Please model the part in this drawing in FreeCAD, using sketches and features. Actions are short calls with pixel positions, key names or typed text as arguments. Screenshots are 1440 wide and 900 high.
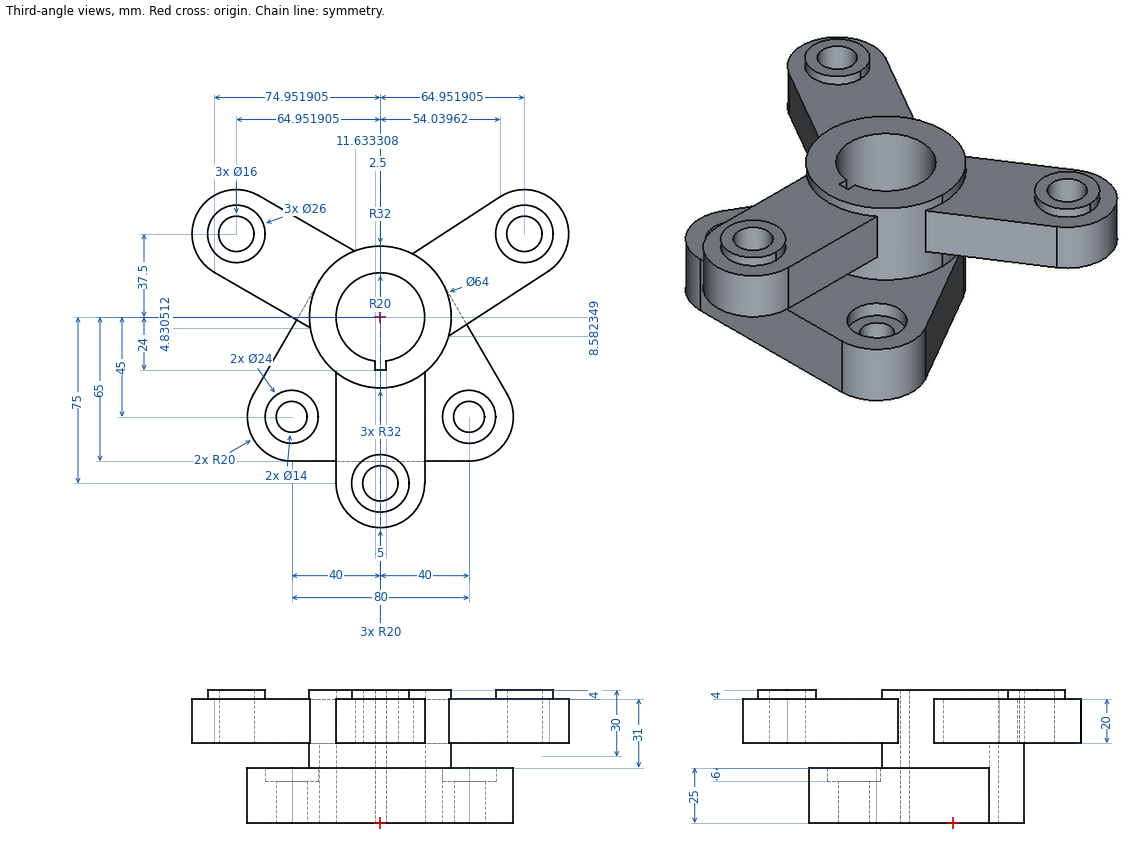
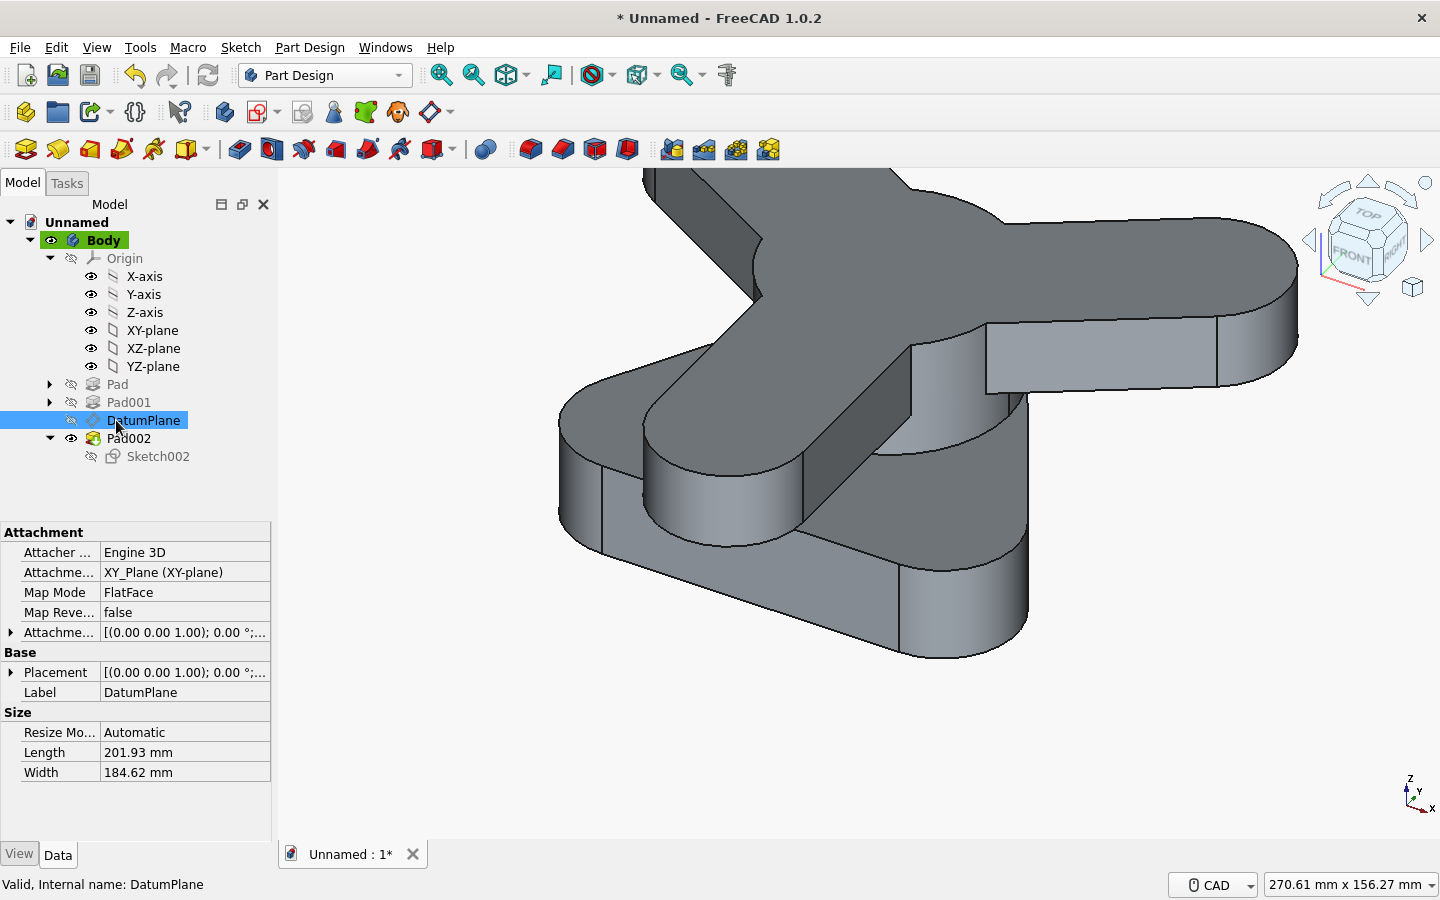
key(v)
key(f)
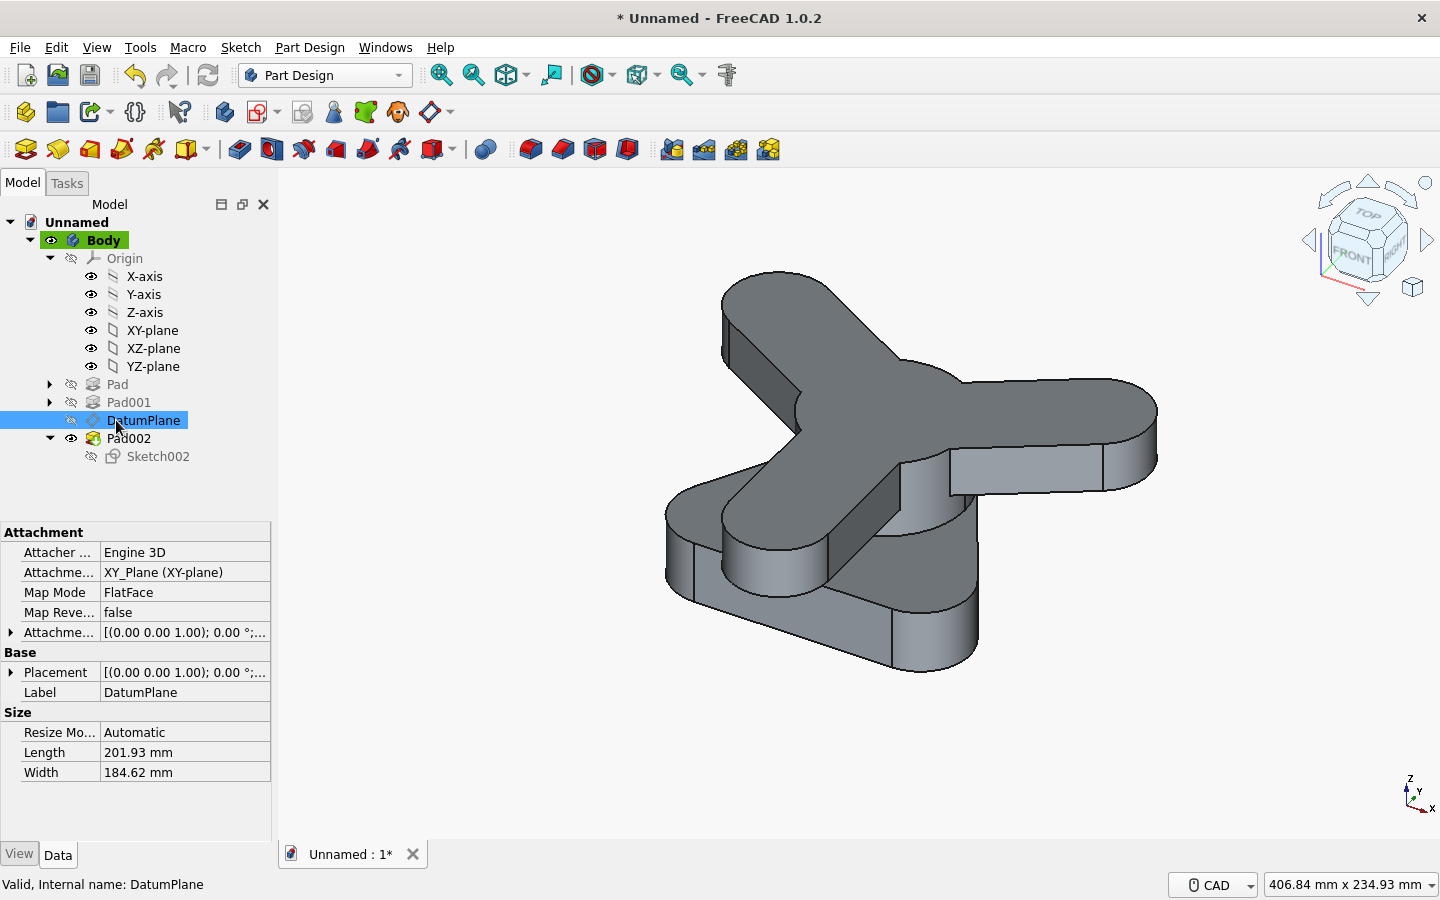
click(890, 406)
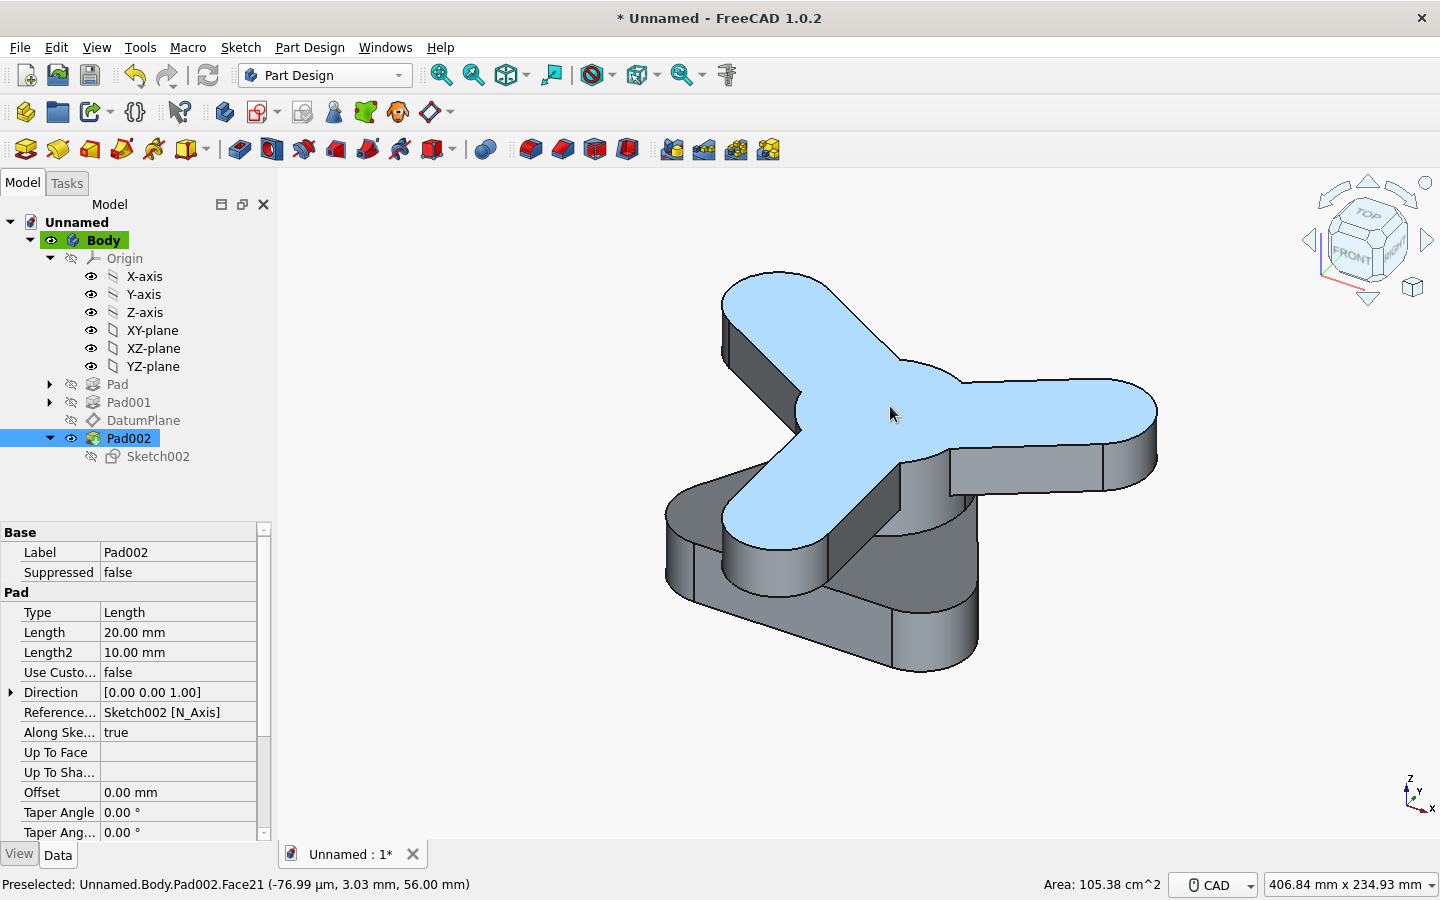
click(258, 112)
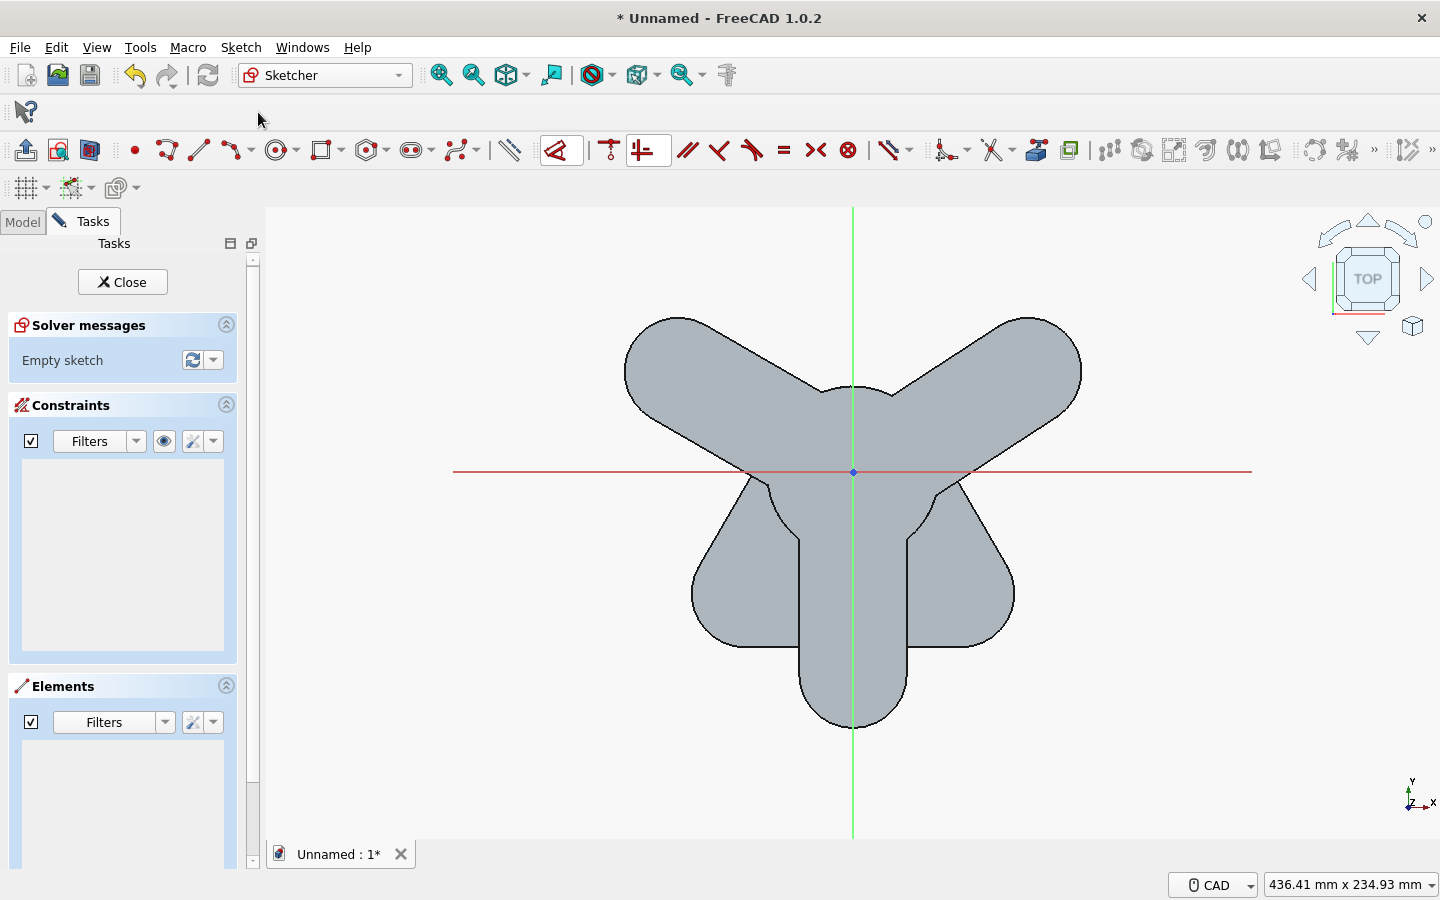
scroll(909, 431, up, 4)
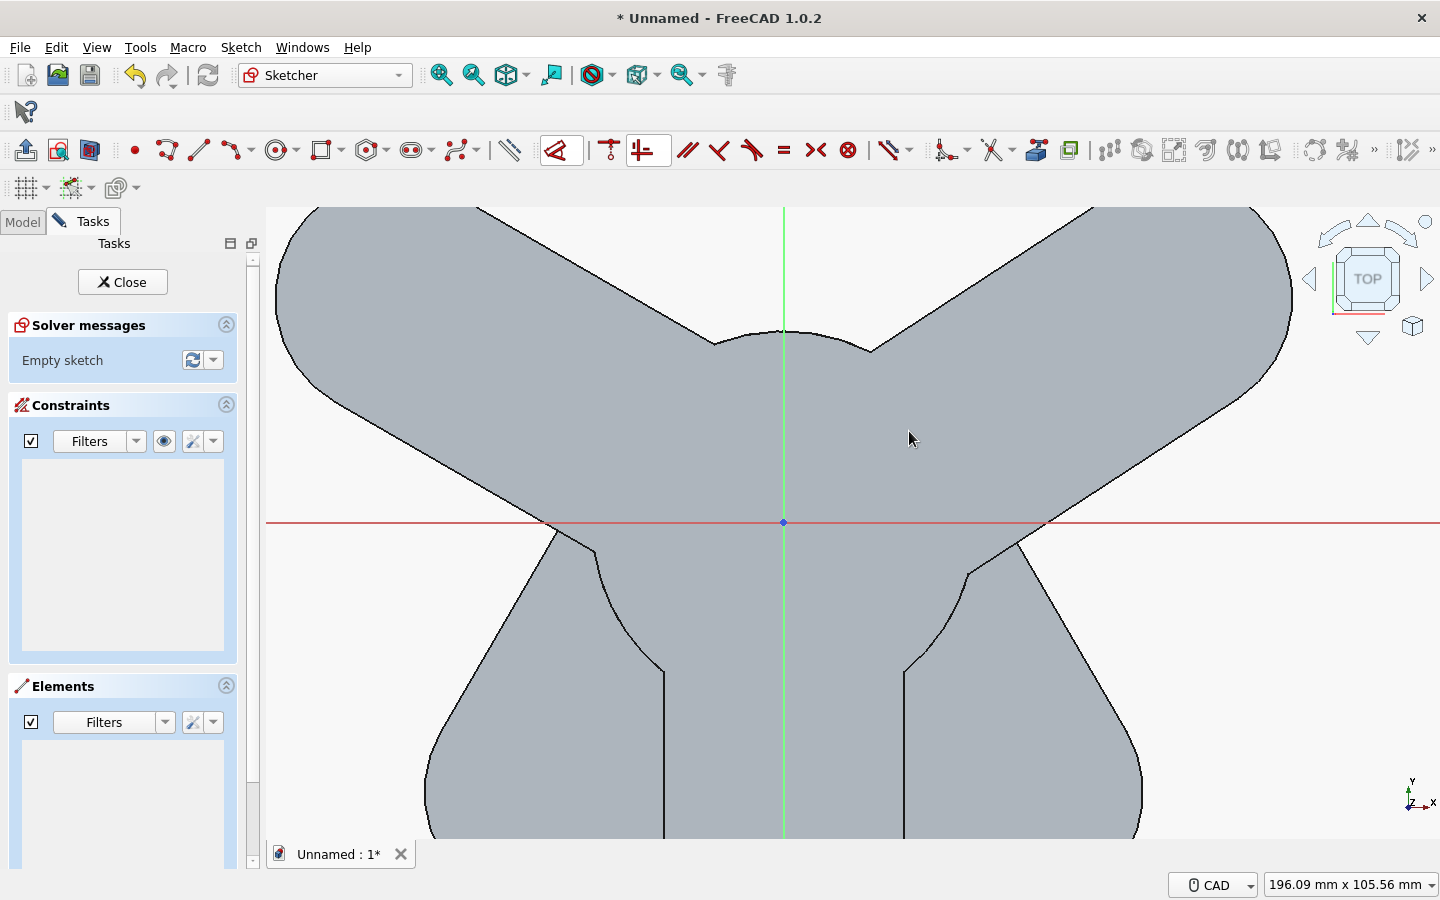
click(276, 150)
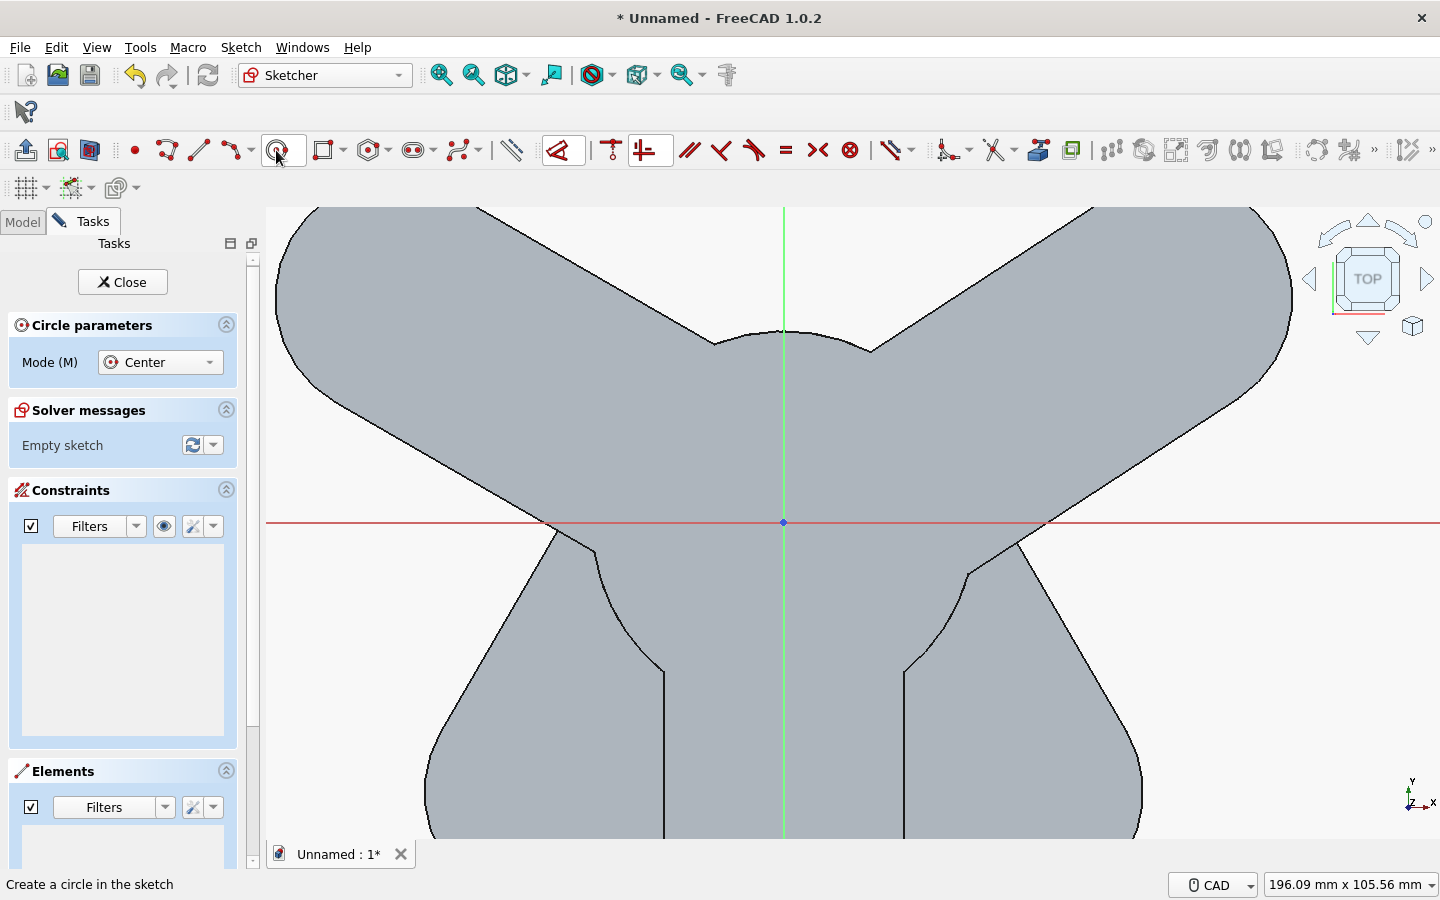
click(784, 523)
move(919, 387)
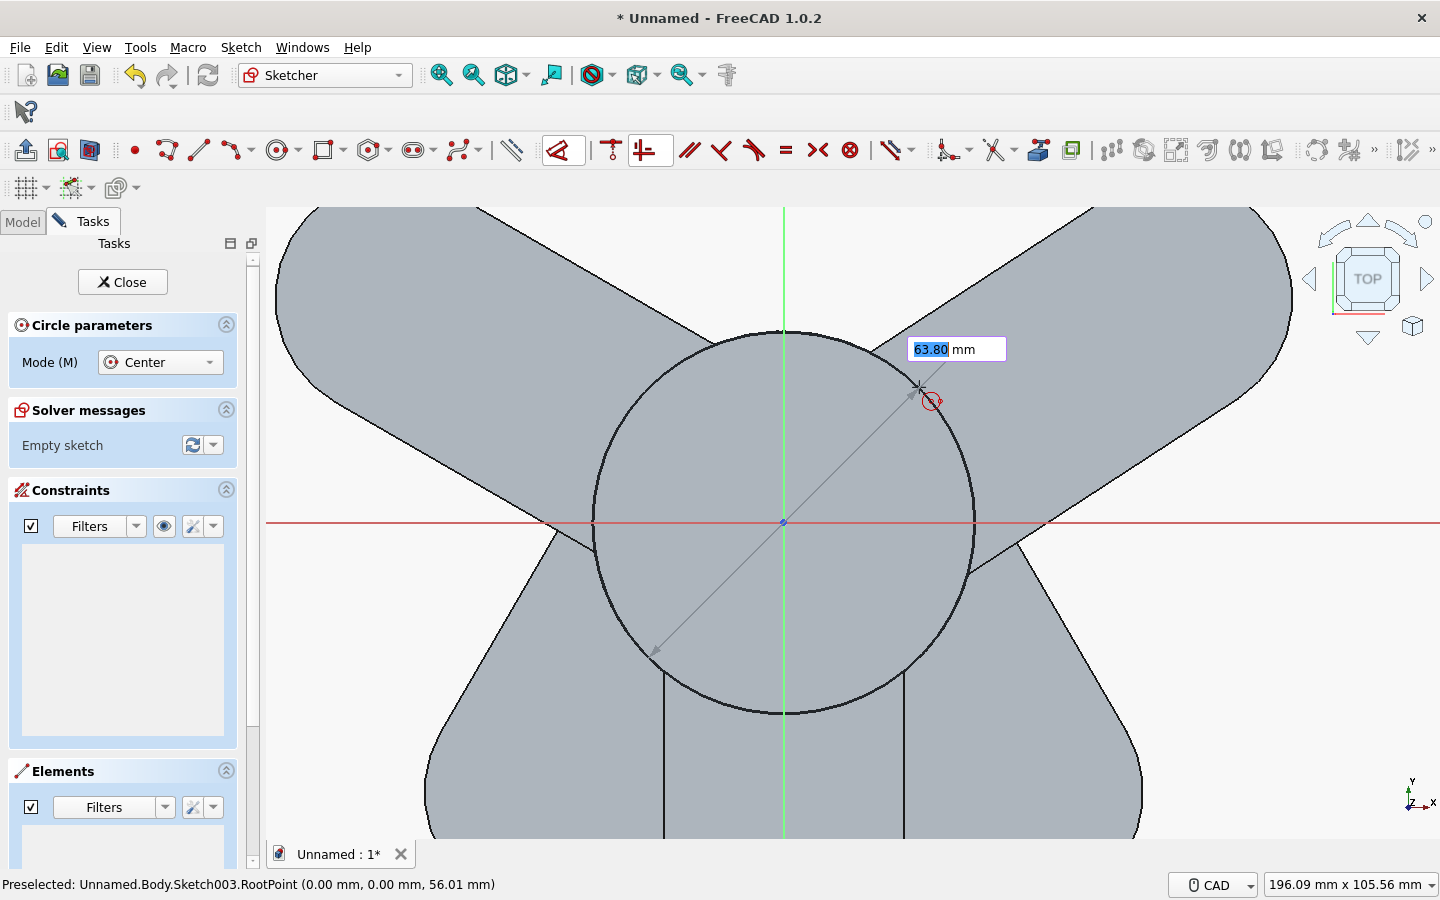
text(64)
key(Return)
key(Escape)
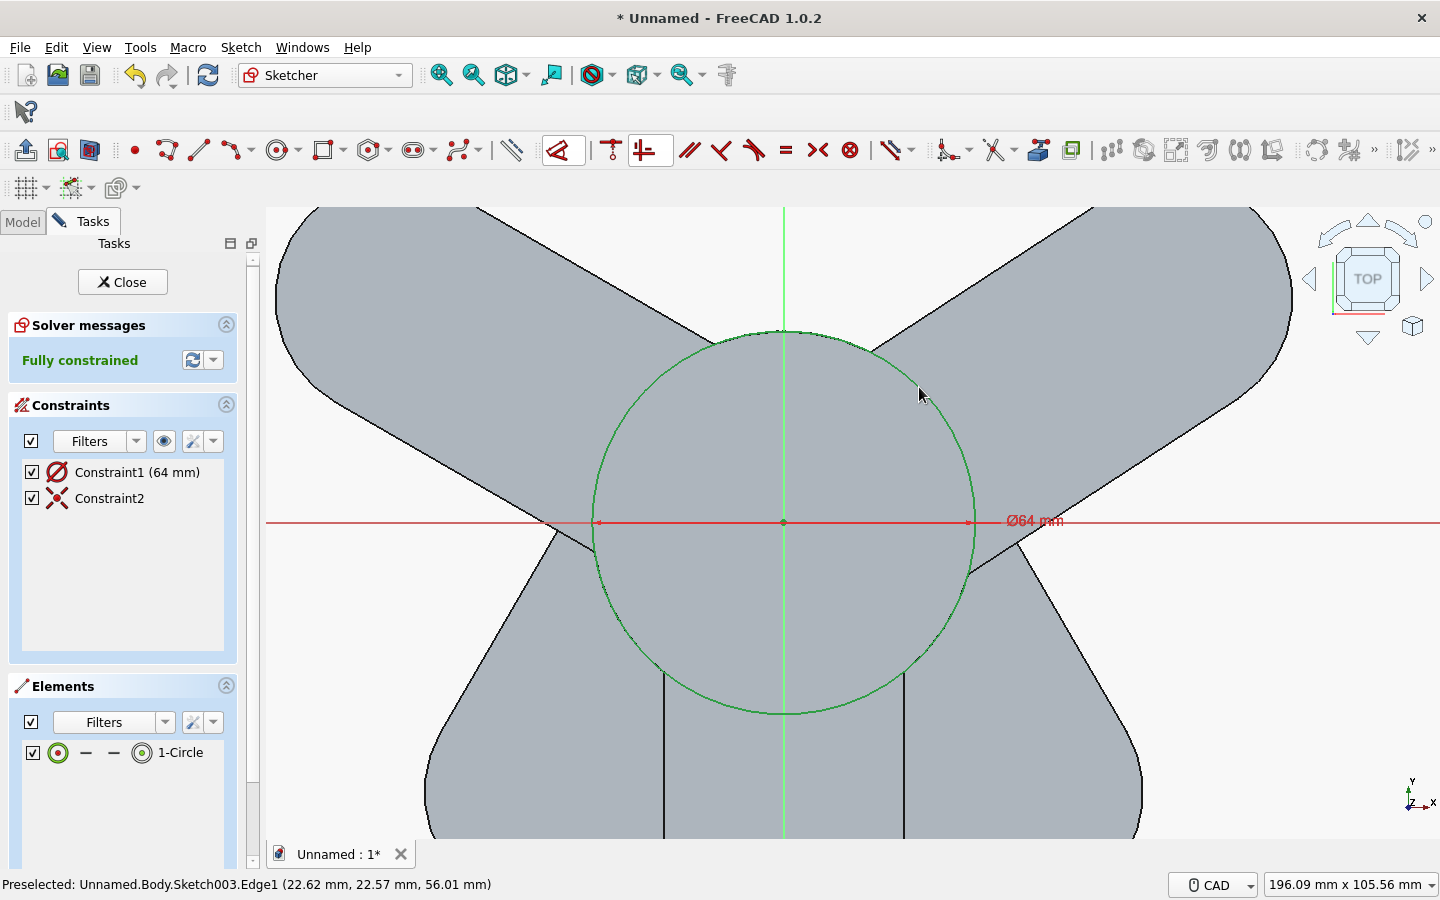
click(123, 282)